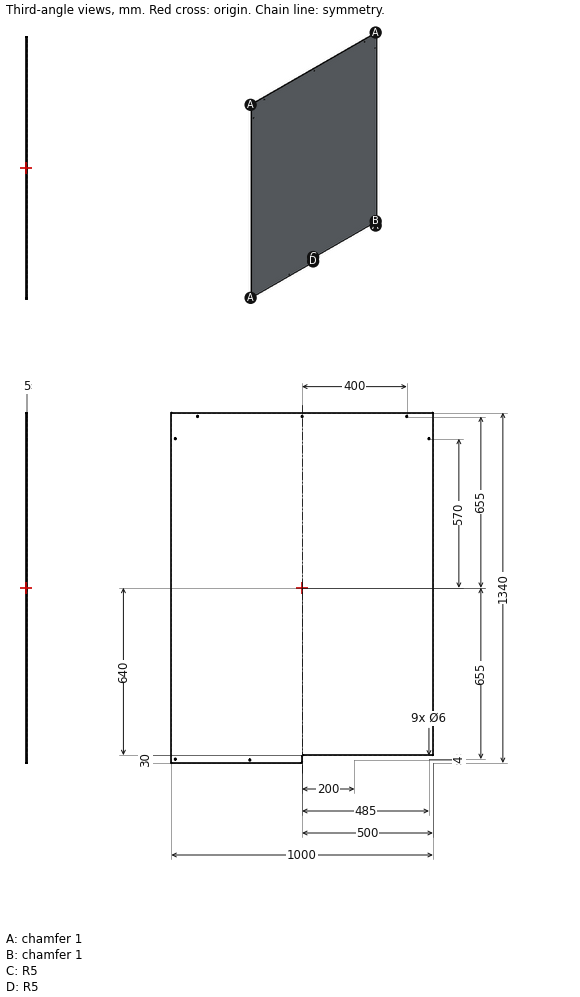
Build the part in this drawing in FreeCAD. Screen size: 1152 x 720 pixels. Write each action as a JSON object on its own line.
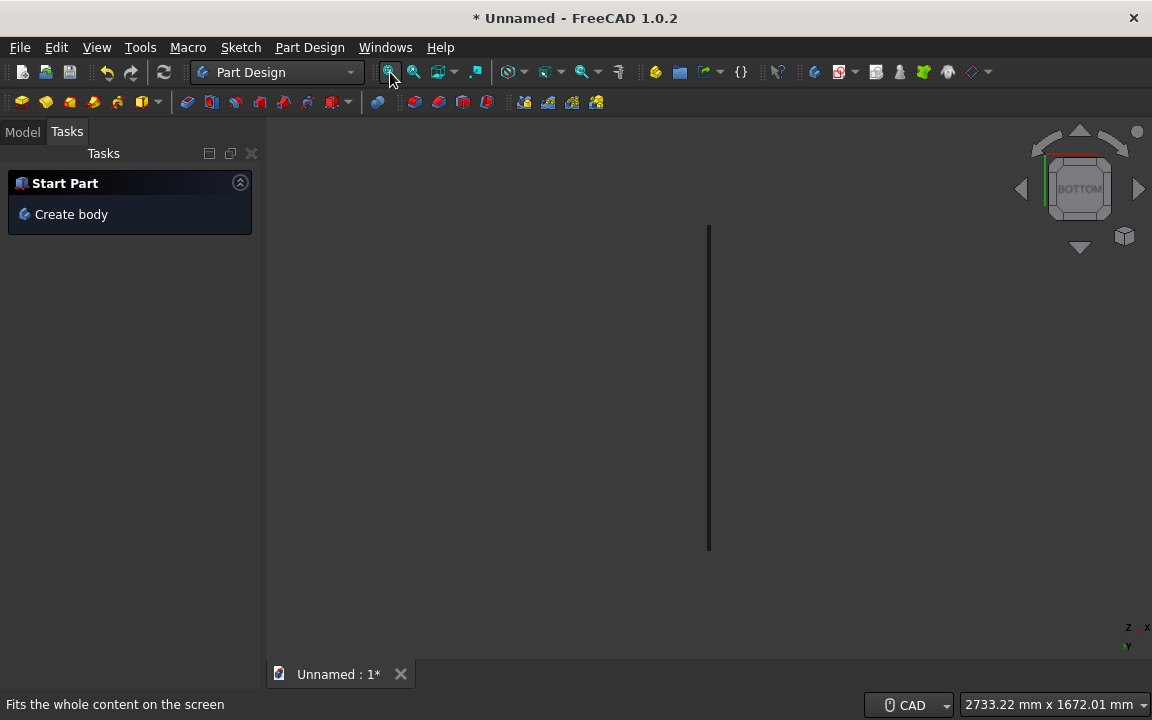
{"action": "scroll", "coordinate": [709, 387], "scroll_direction": "up", "scroll_amount": 15}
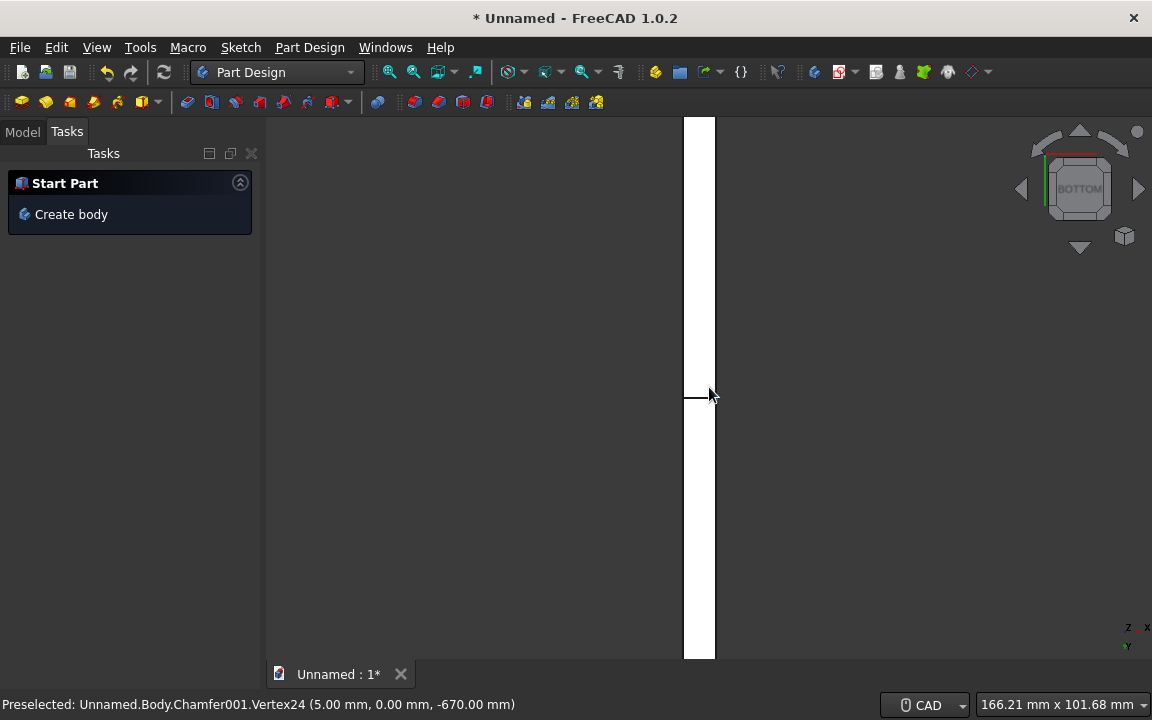
{"action": "left_click", "coordinate": [390, 72]}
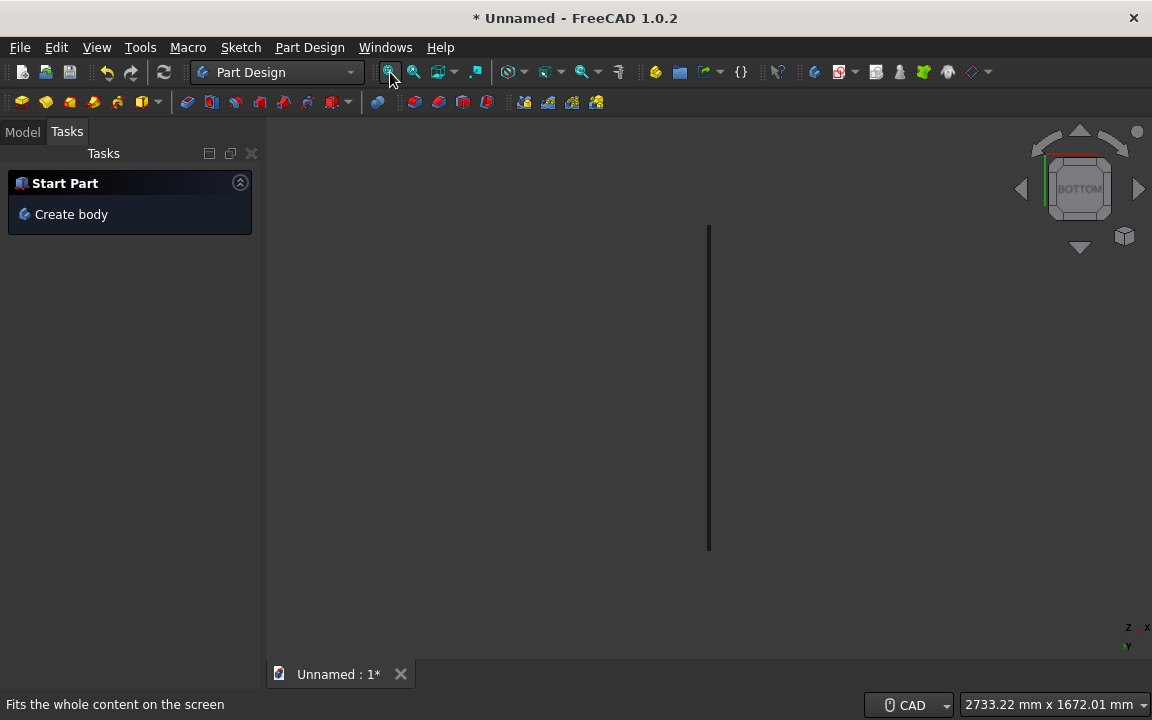
{"action": "key", "text": "4"}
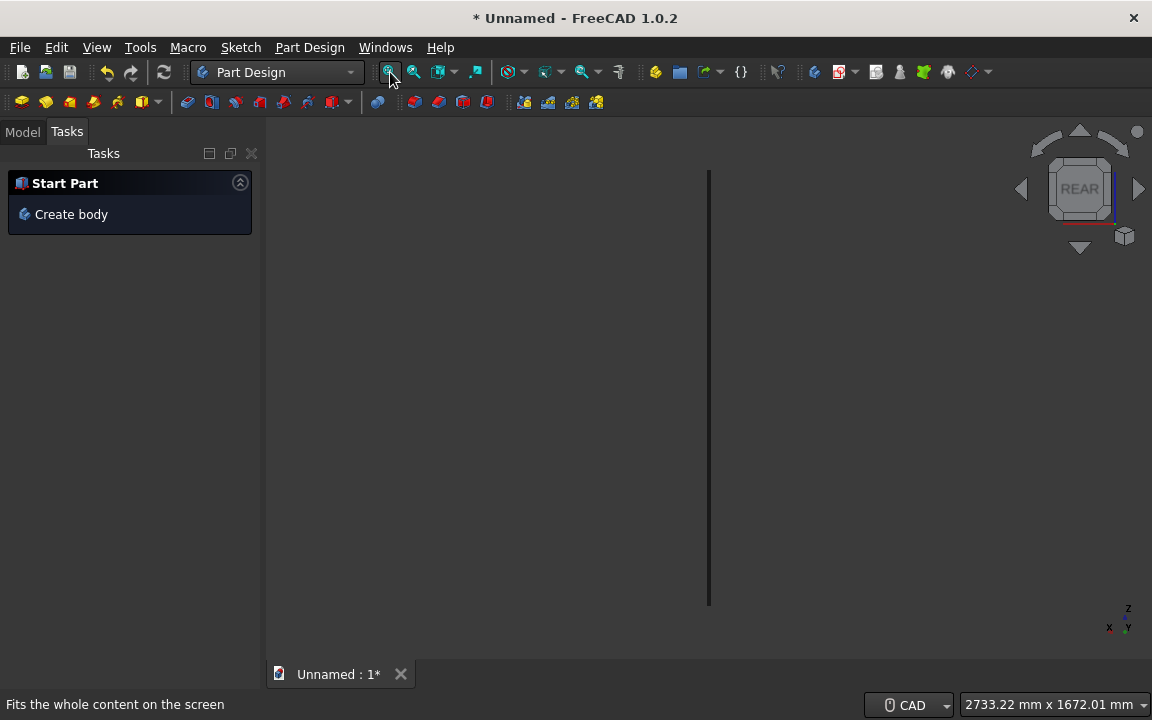
{"action": "scroll", "coordinate": [709, 594], "scroll_direction": "up", "scroll_amount": 15}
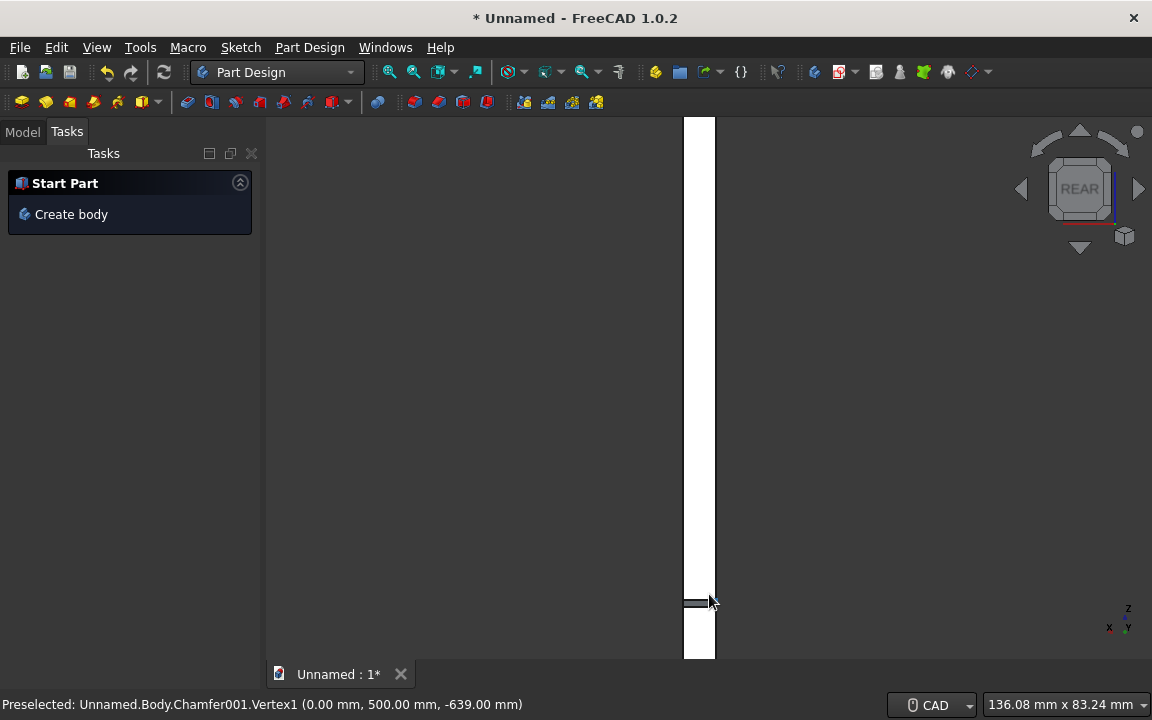
{"action": "left_click", "coordinate": [390, 72]}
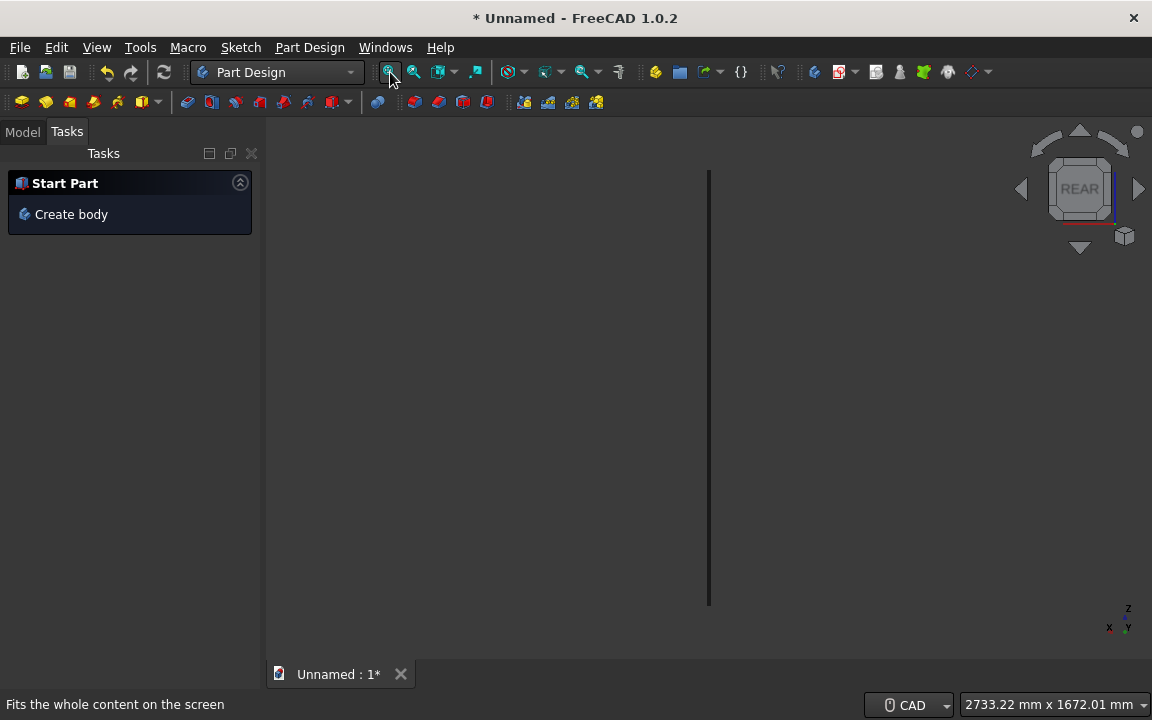
{"action": "key", "text": "6"}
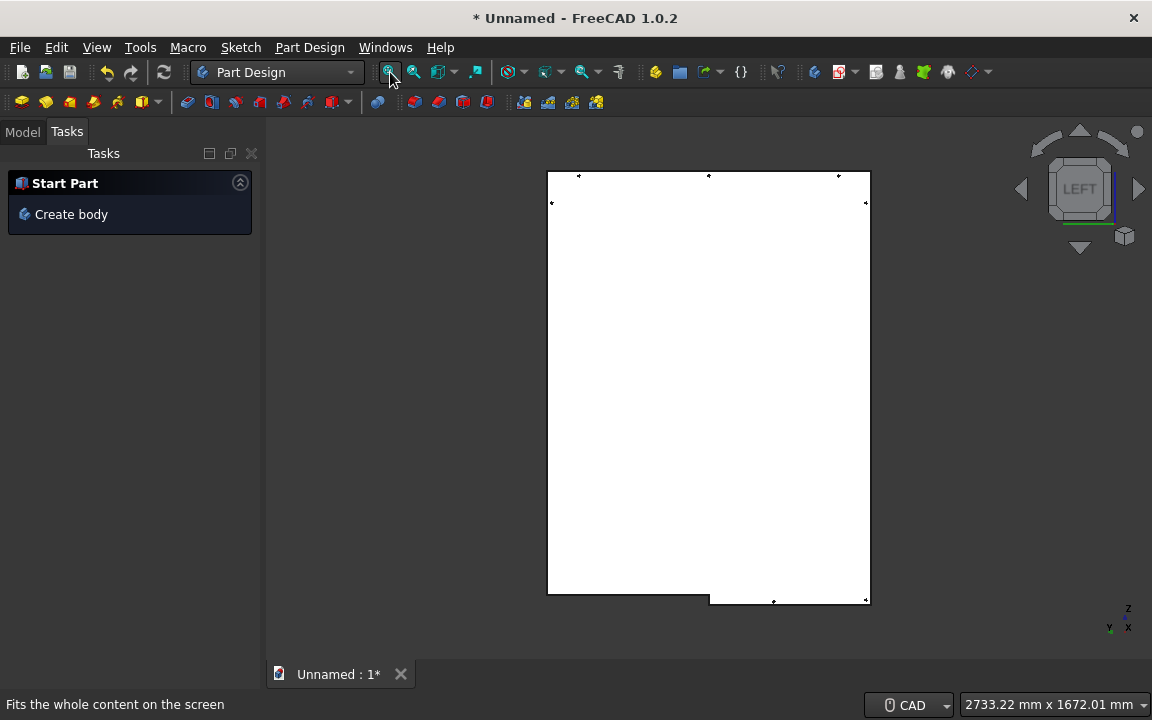
{"action": "scroll", "coordinate": [709, 594], "scroll_direction": "up", "scroll_amount": 15}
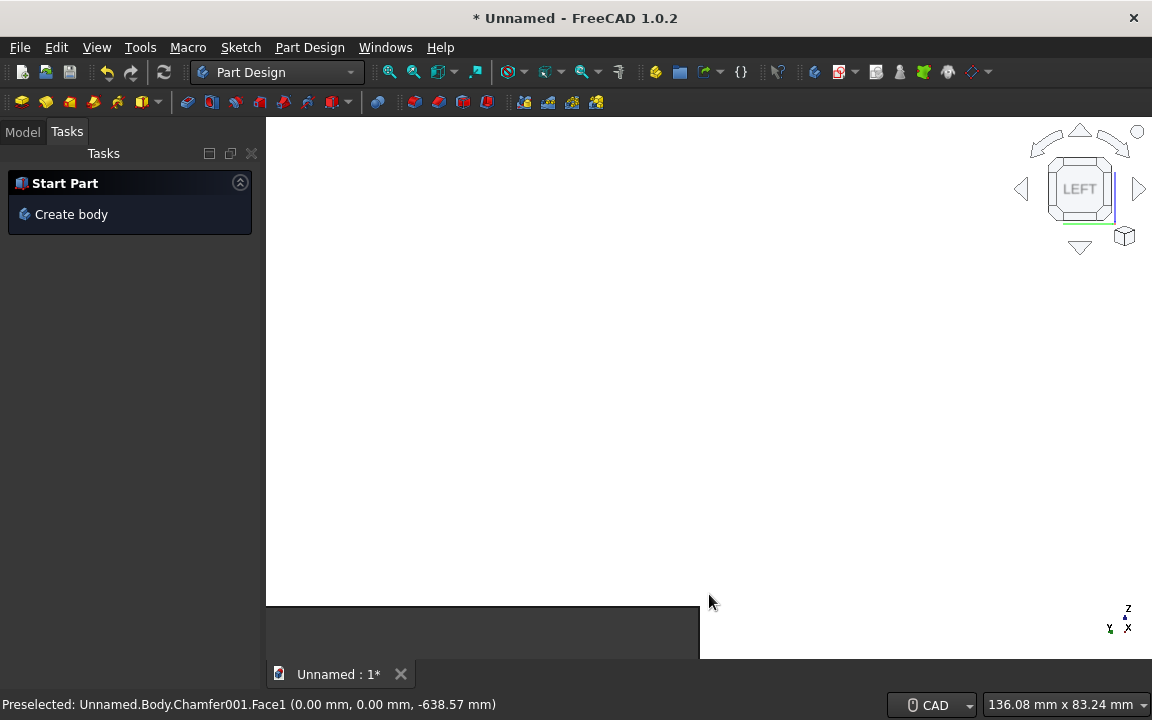
{"action": "left_click", "coordinate": [390, 72]}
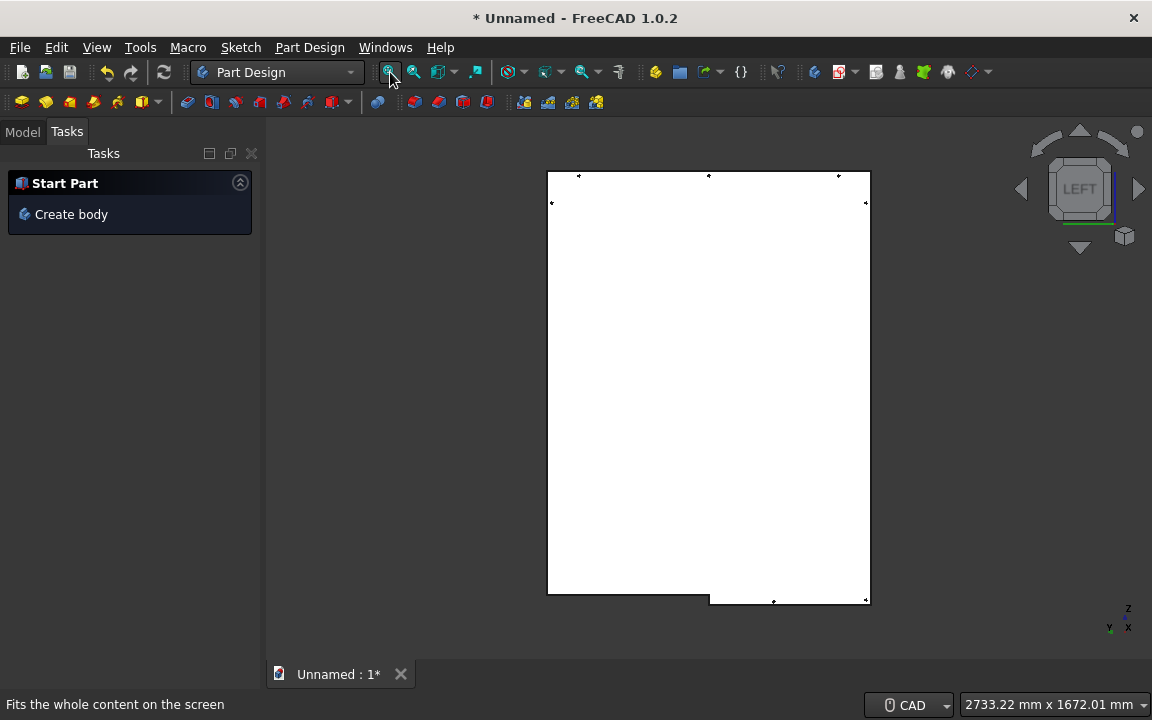
{"action": "key", "text": "v 3"}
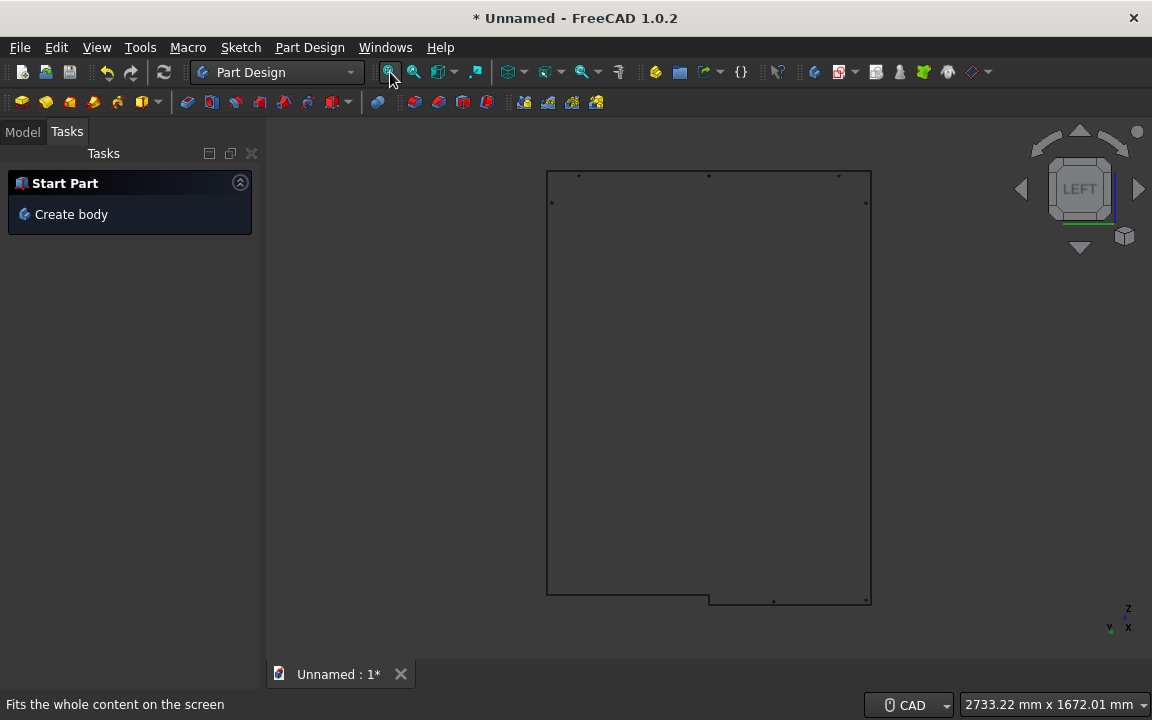
{"action": "key", "text": "0"}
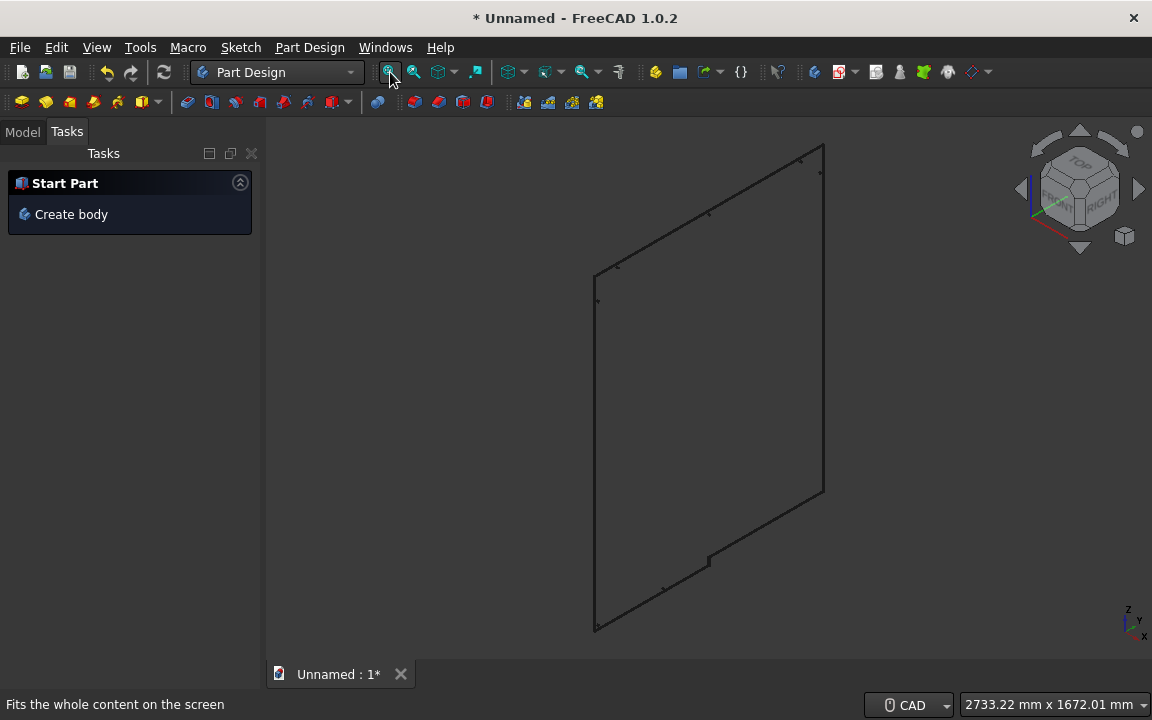
{"action": "scroll", "coordinate": [709, 556], "scroll_direction": "up", "scroll_amount": 15}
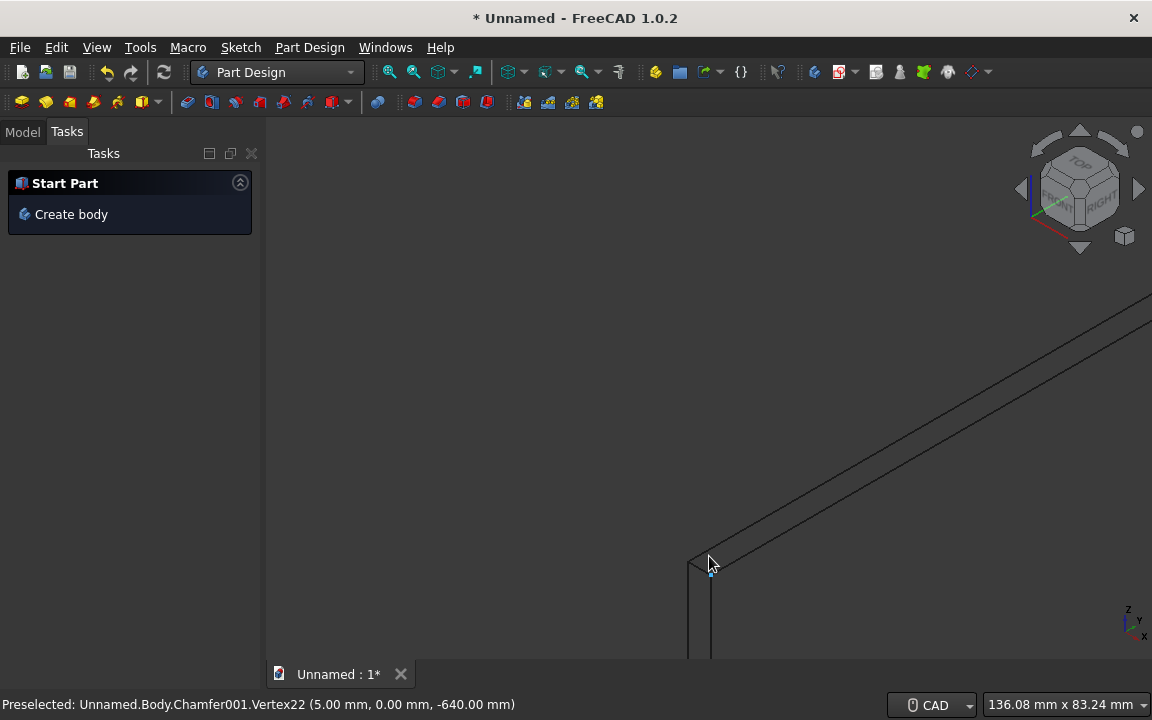
{"action": "left_click", "coordinate": [699, 567]}